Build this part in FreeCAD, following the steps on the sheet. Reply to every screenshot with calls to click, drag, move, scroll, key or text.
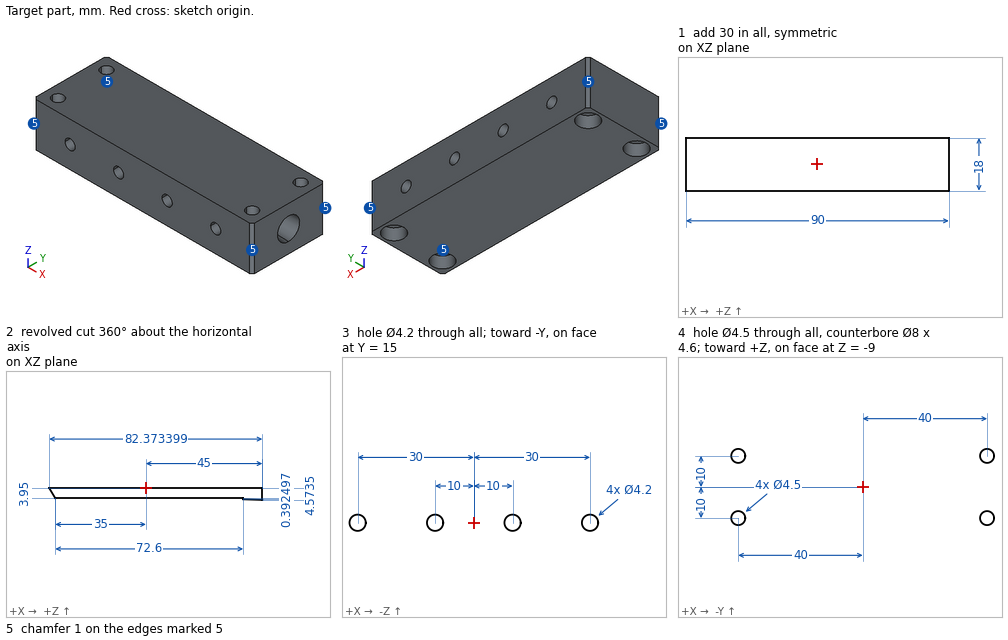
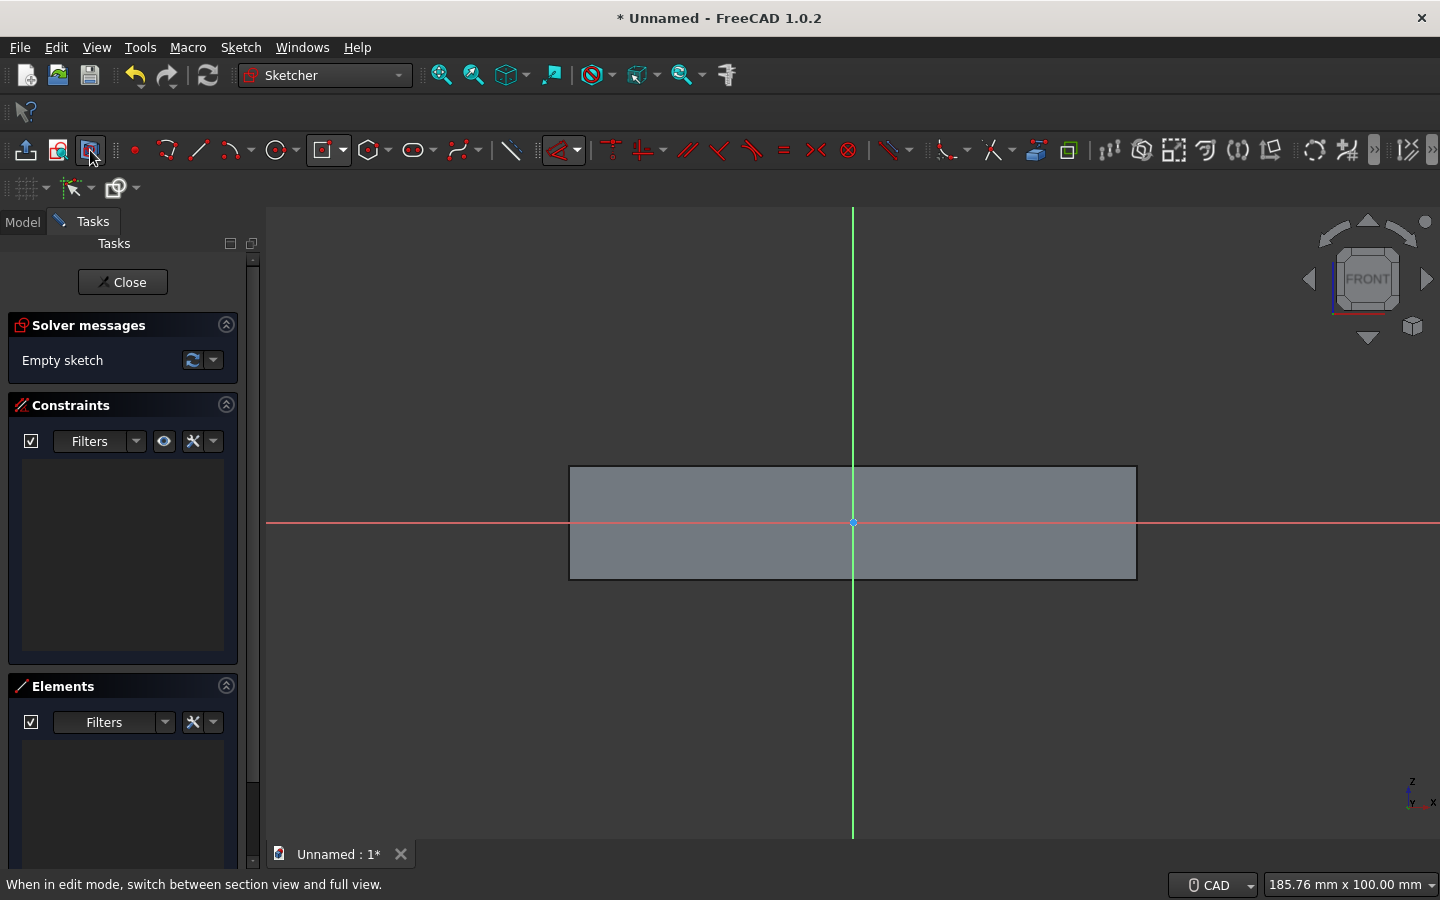
click(168, 150)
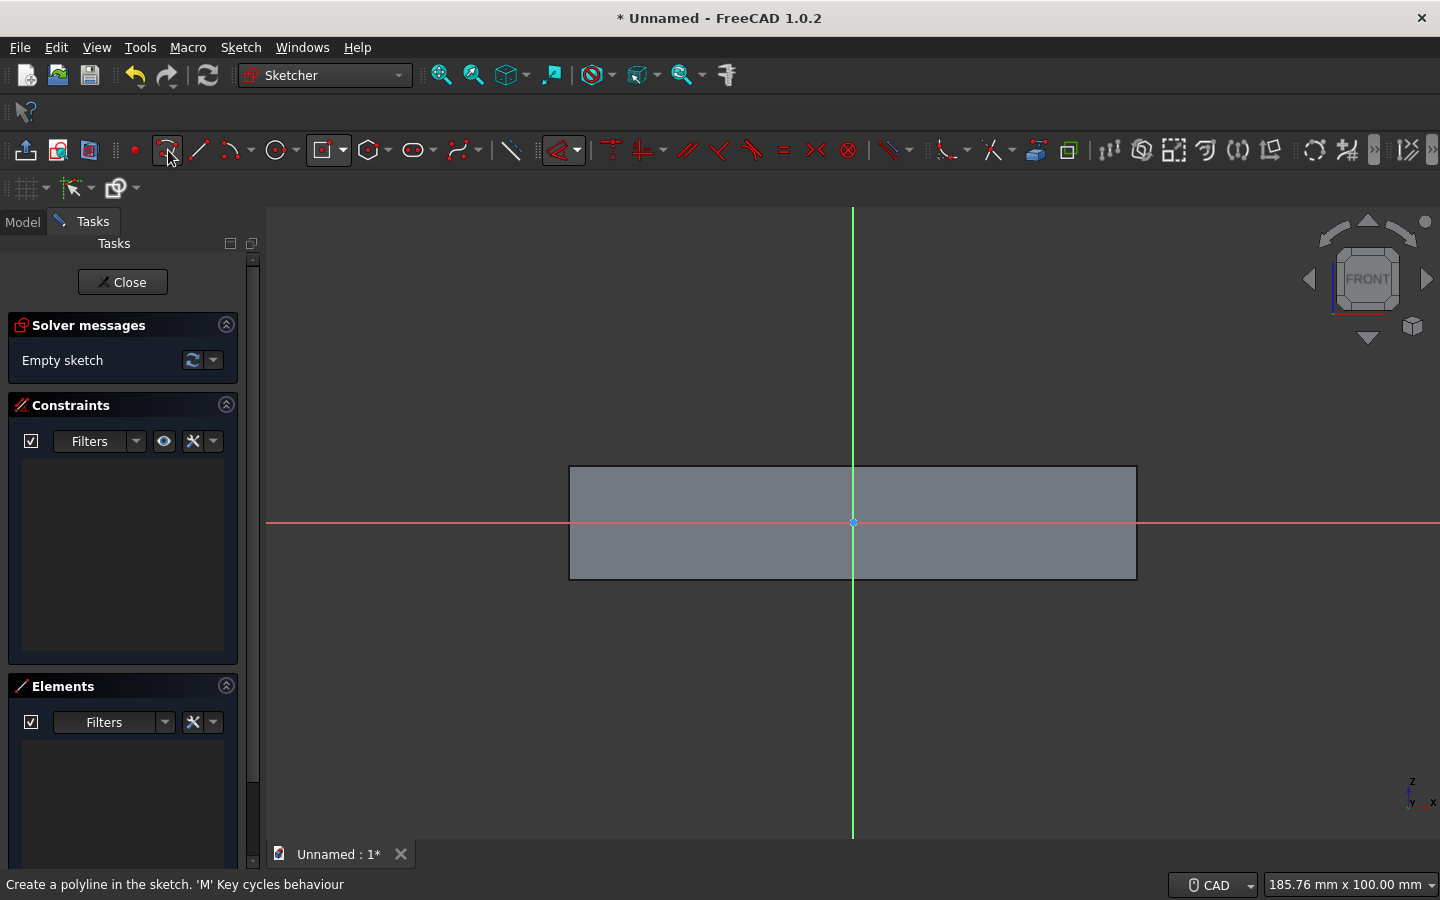
click(632, 548)
click(617, 523)
click(1137, 532)
click(1137, 552)
click(1091, 548)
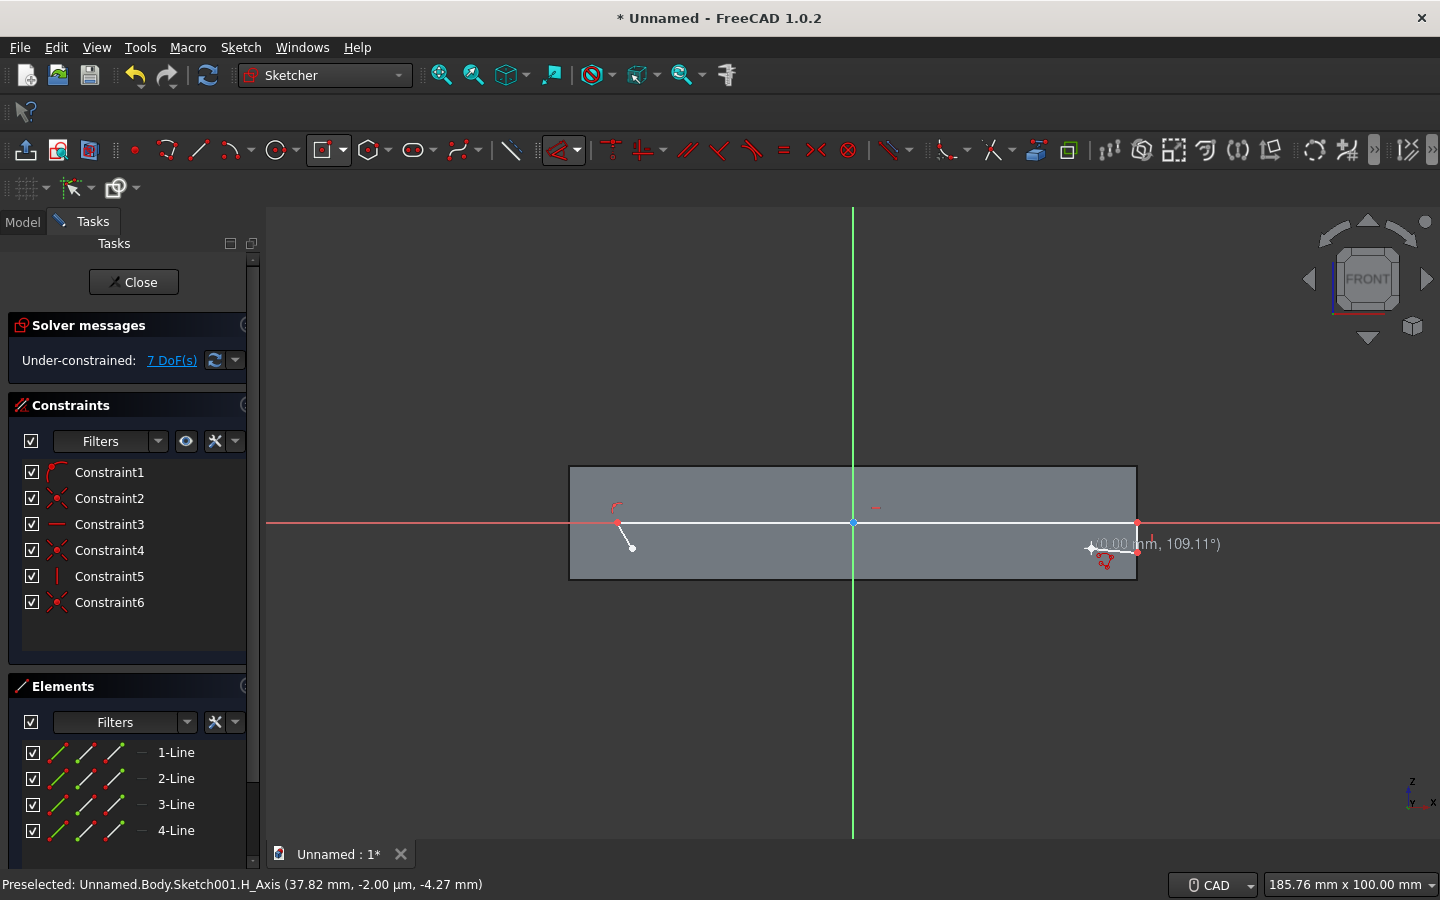
scroll(1091, 548, up, 10)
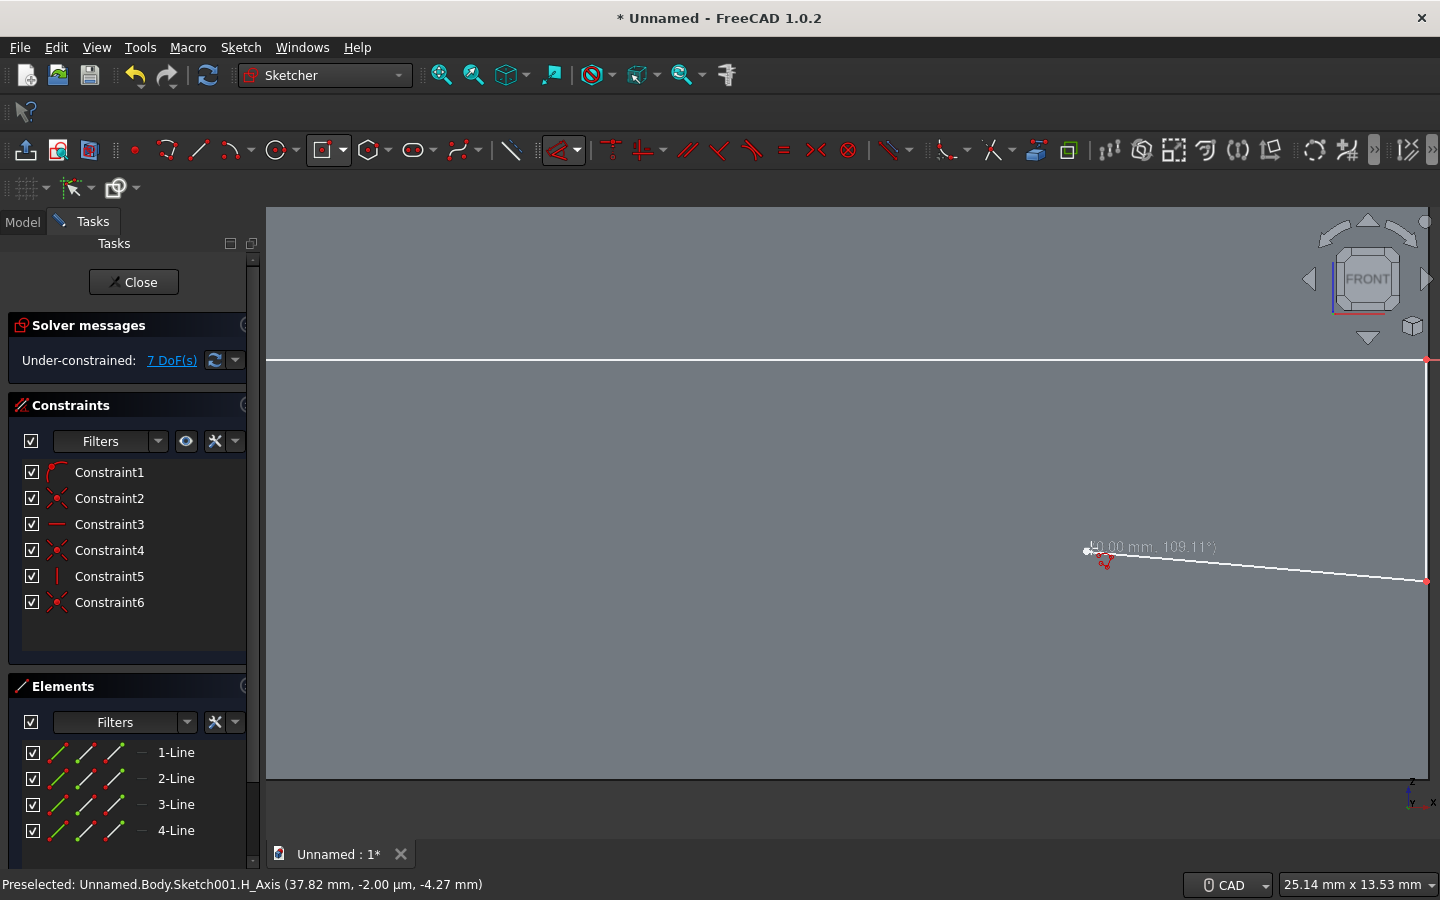
click(1087, 544)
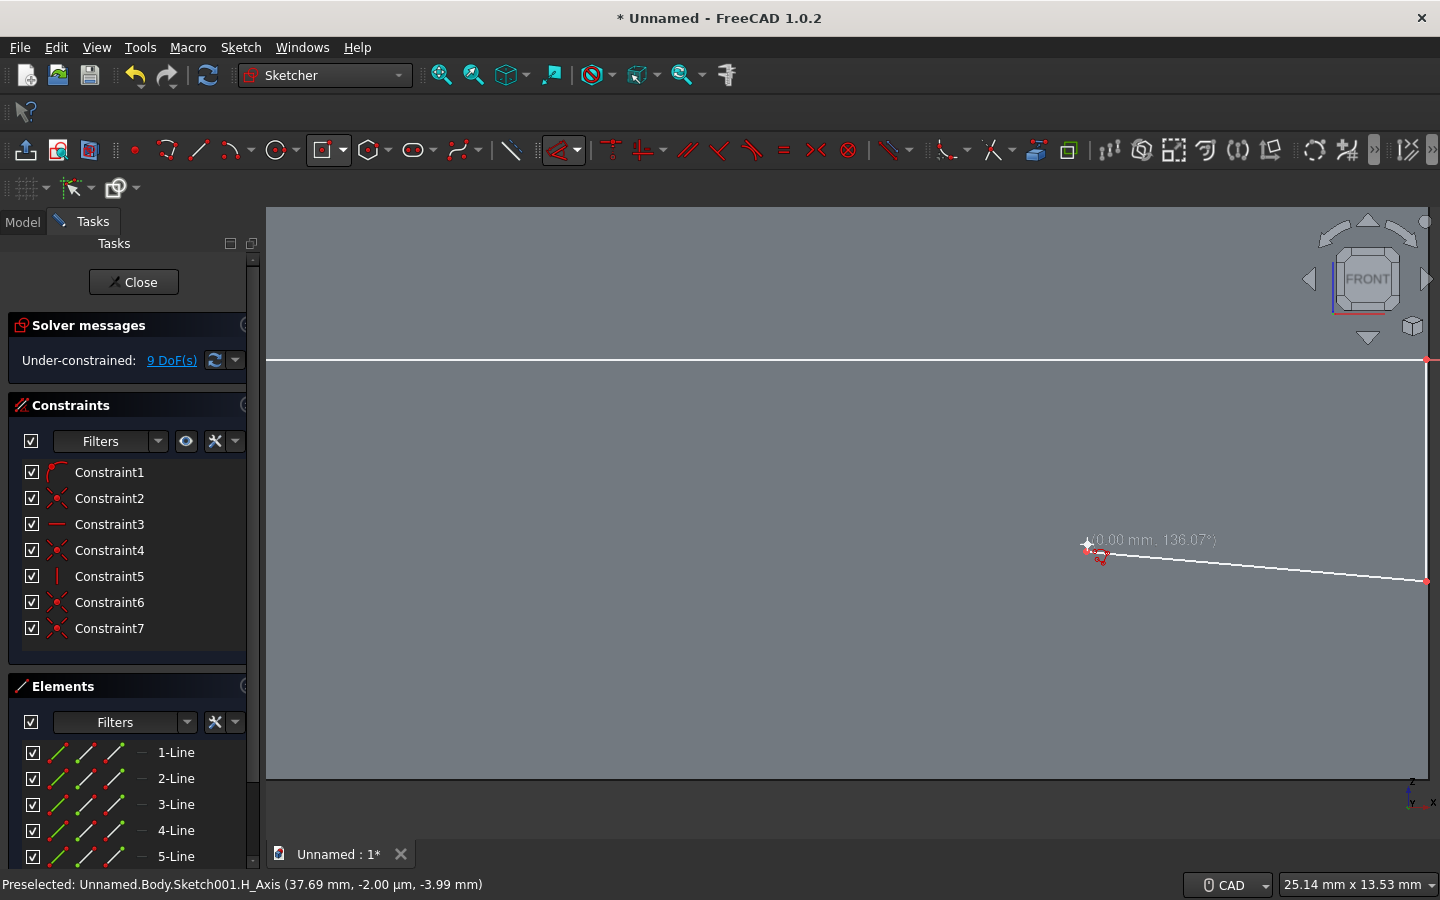
scroll(1038, 534, down, 9)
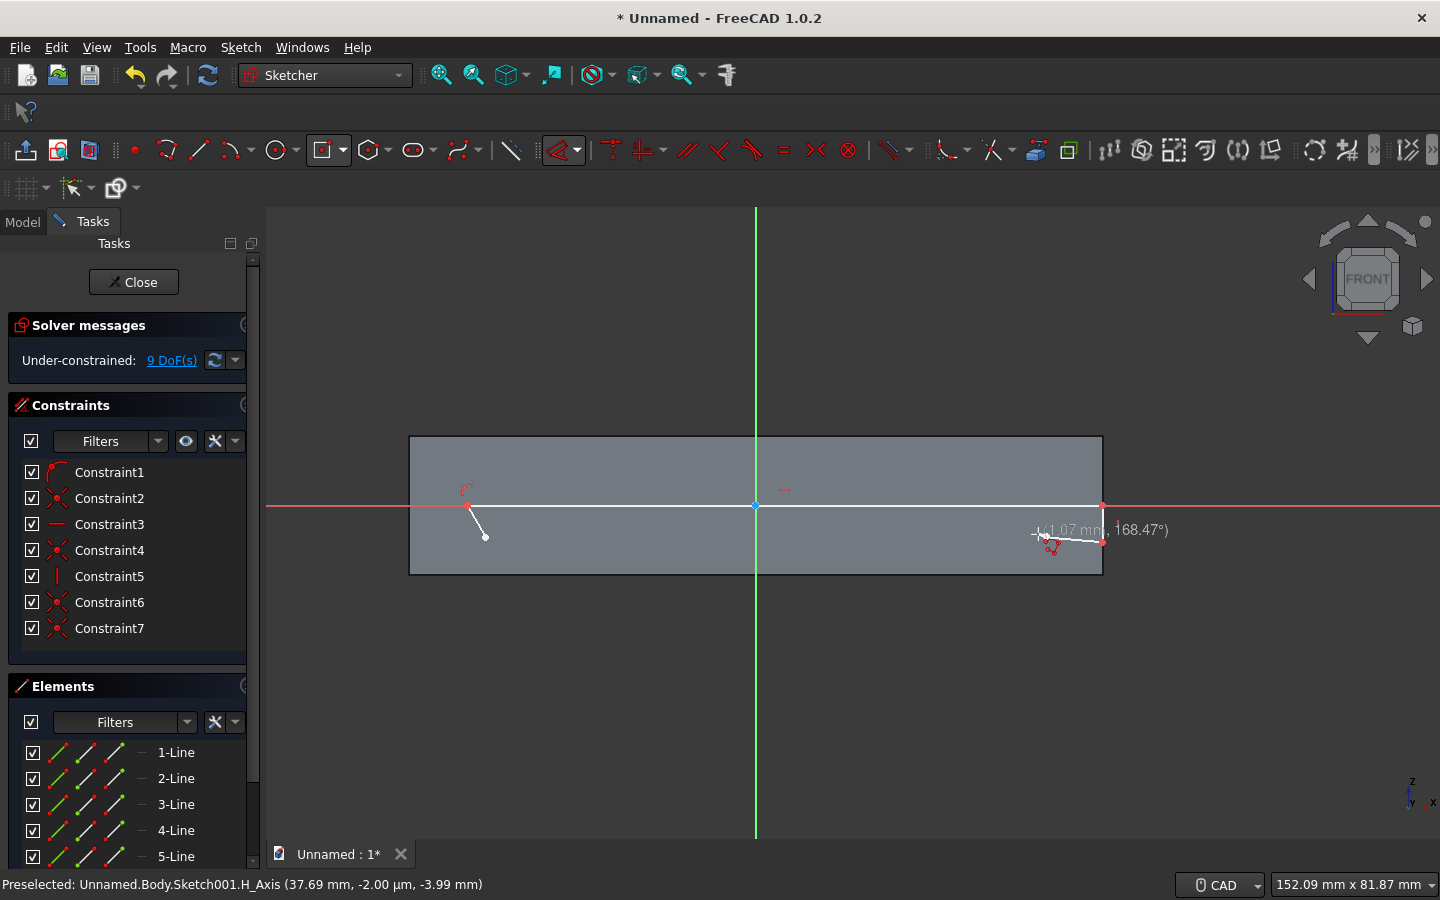
click(486, 537)
key(Escape)
key(Escape)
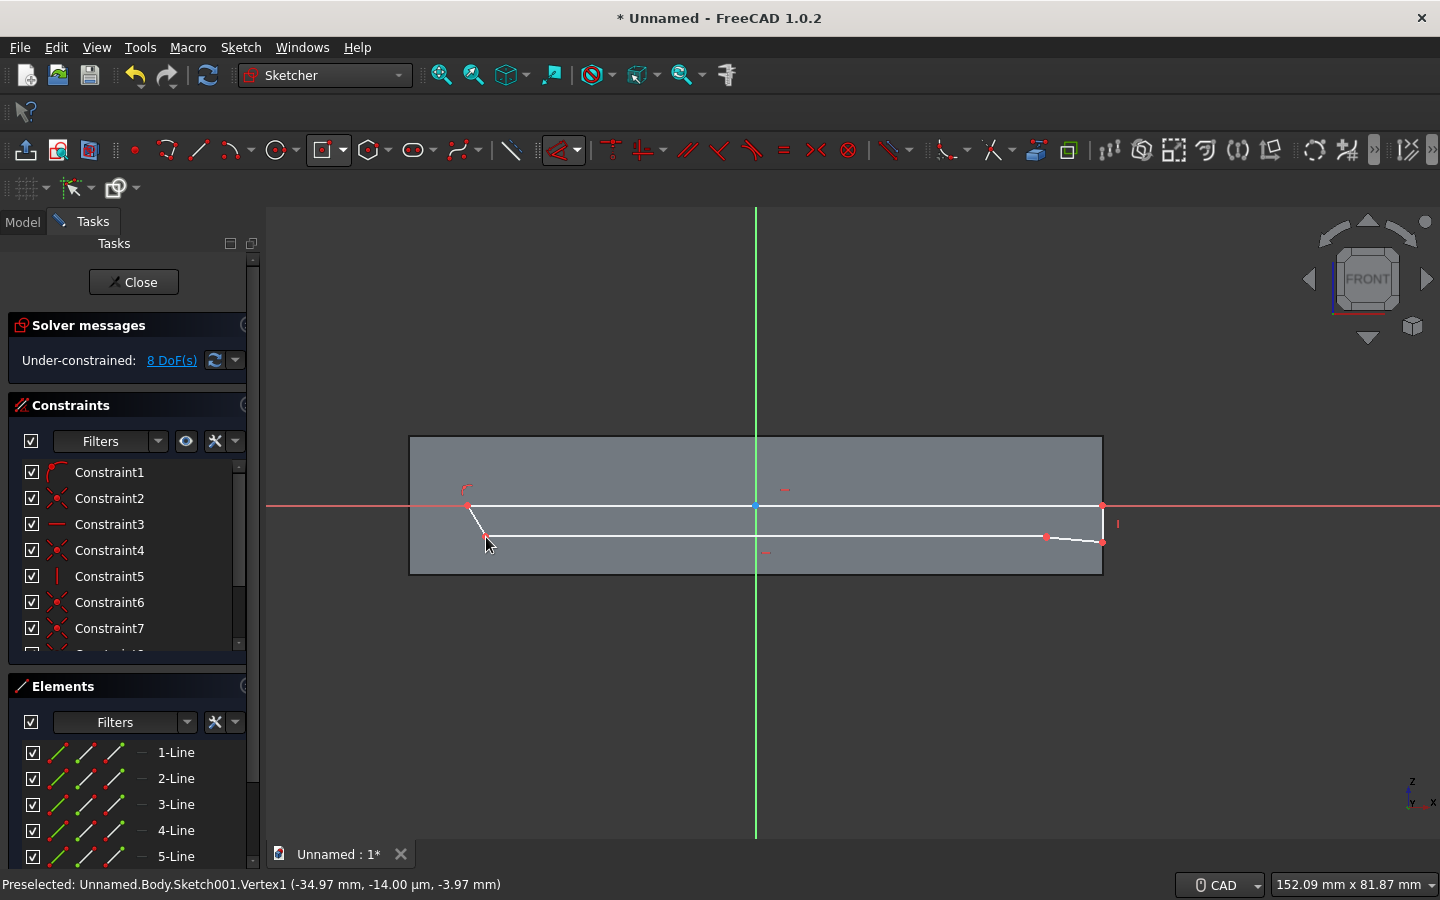
scroll(1047, 537, up, 13)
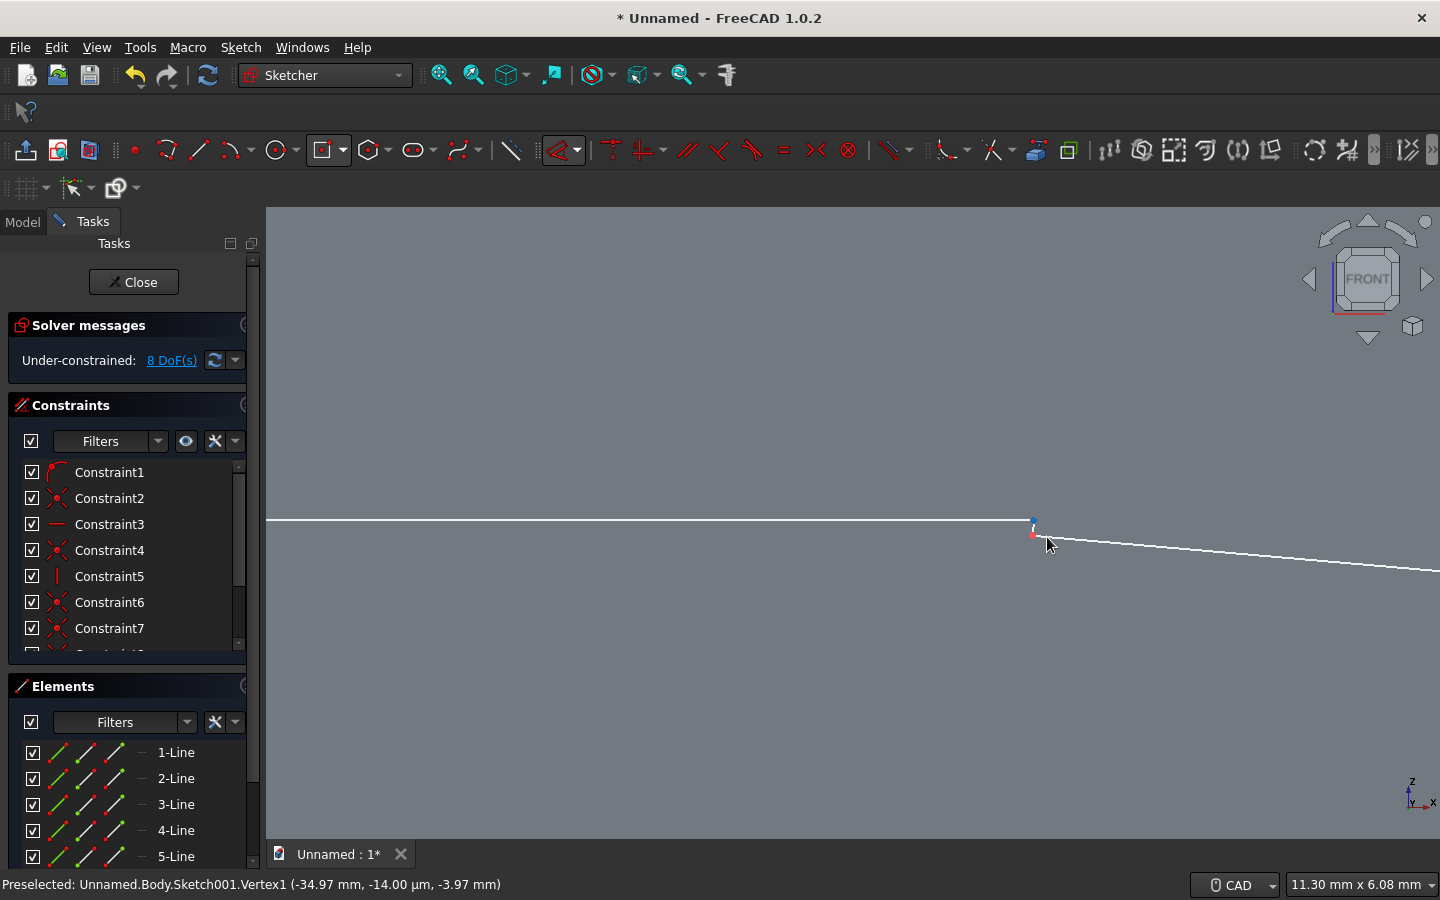
click(1033, 528)